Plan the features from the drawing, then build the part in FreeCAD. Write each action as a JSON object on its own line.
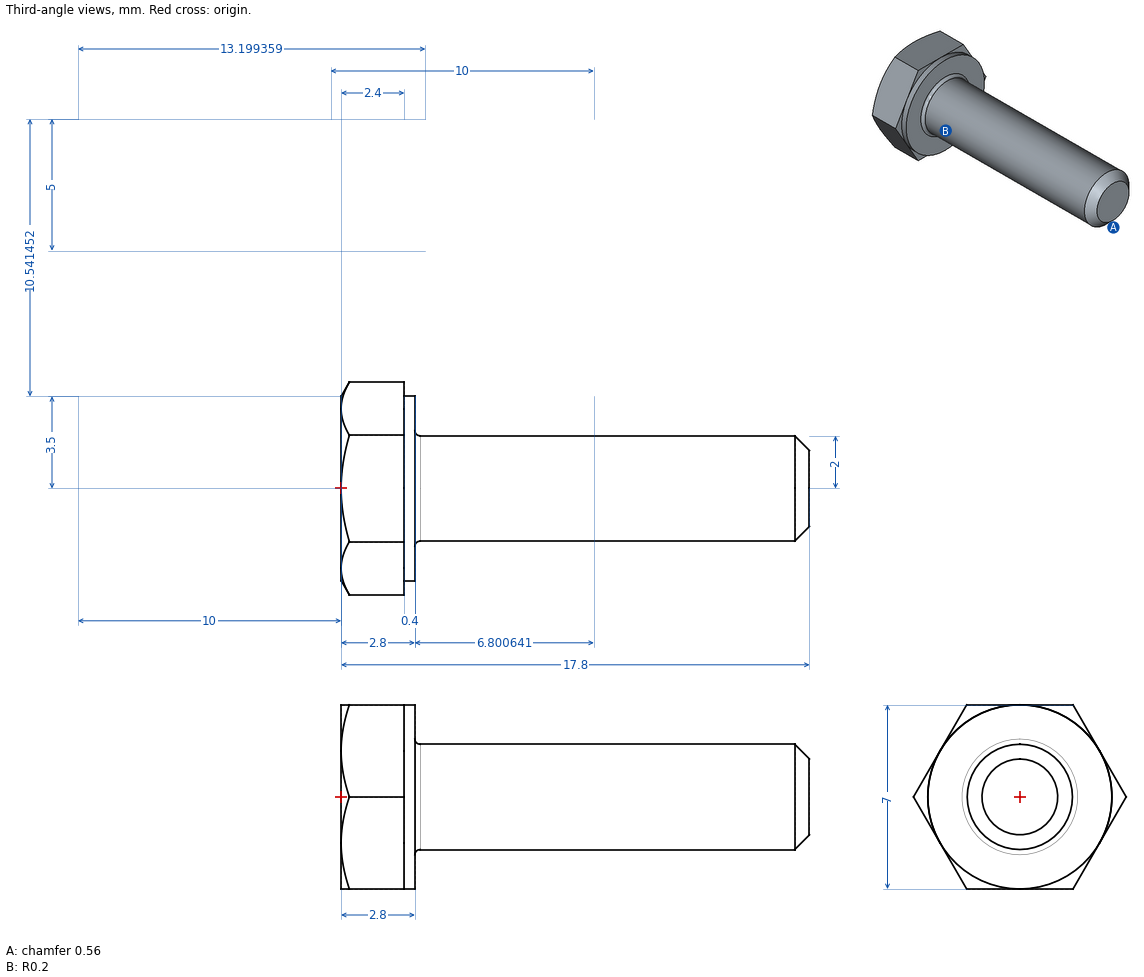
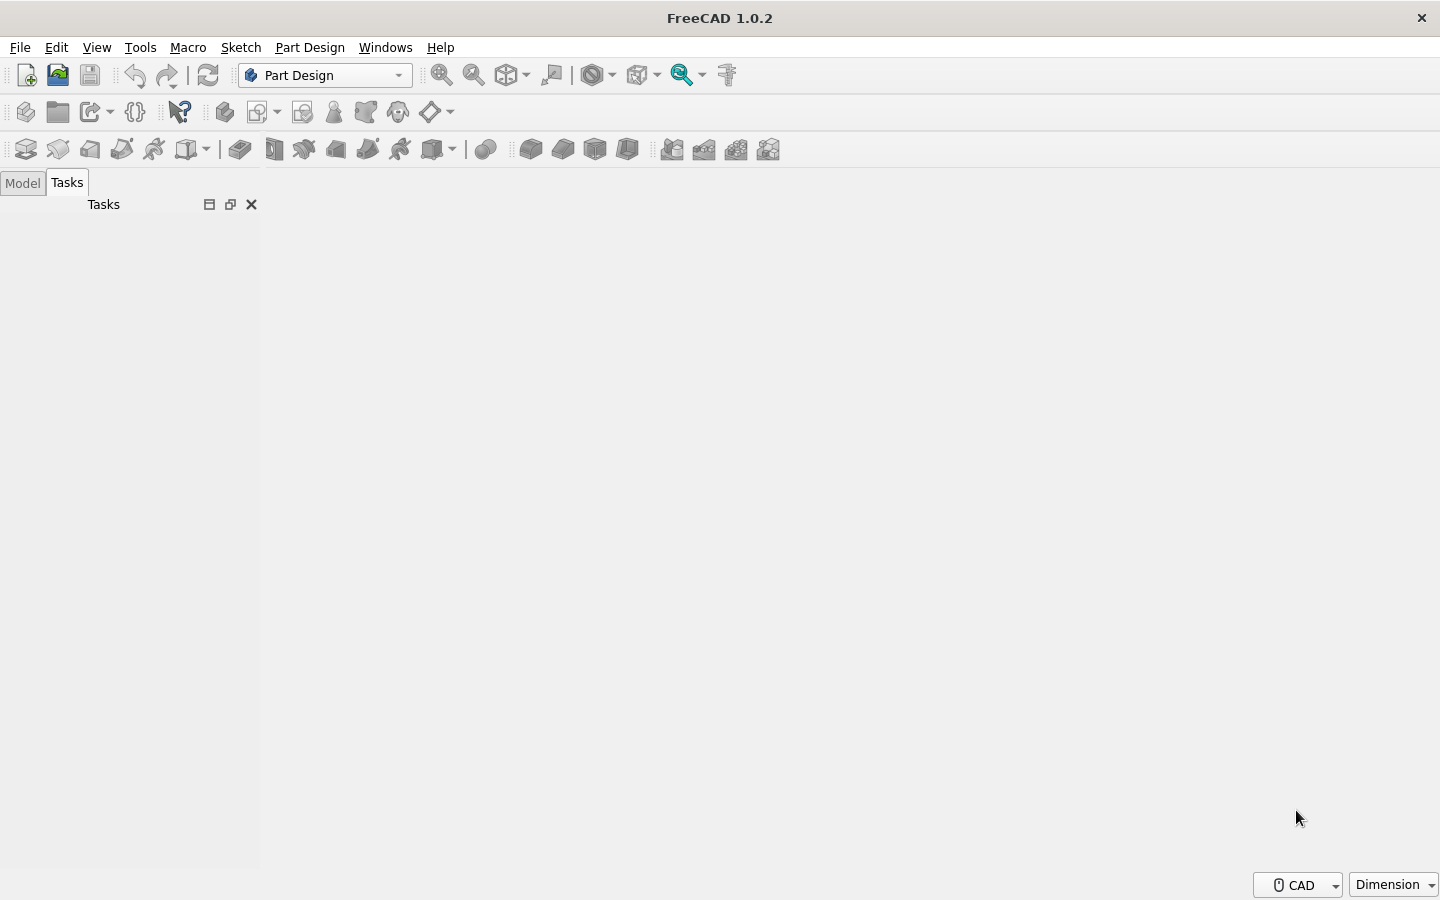
{"action": "key", "text": "ctrl+n"}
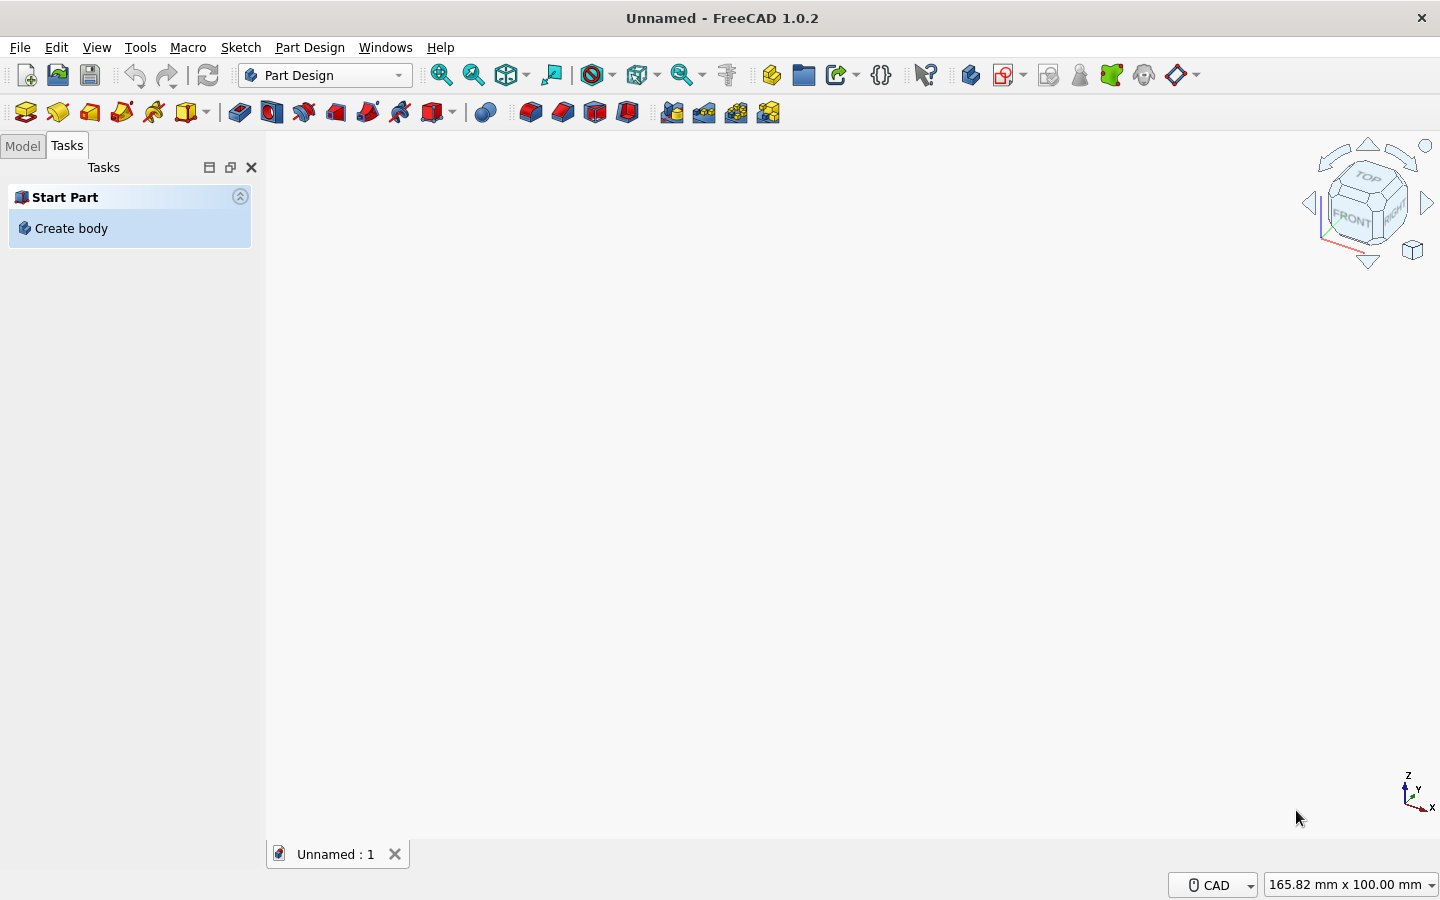
{"action": "left_click", "coordinate": [1004, 76]}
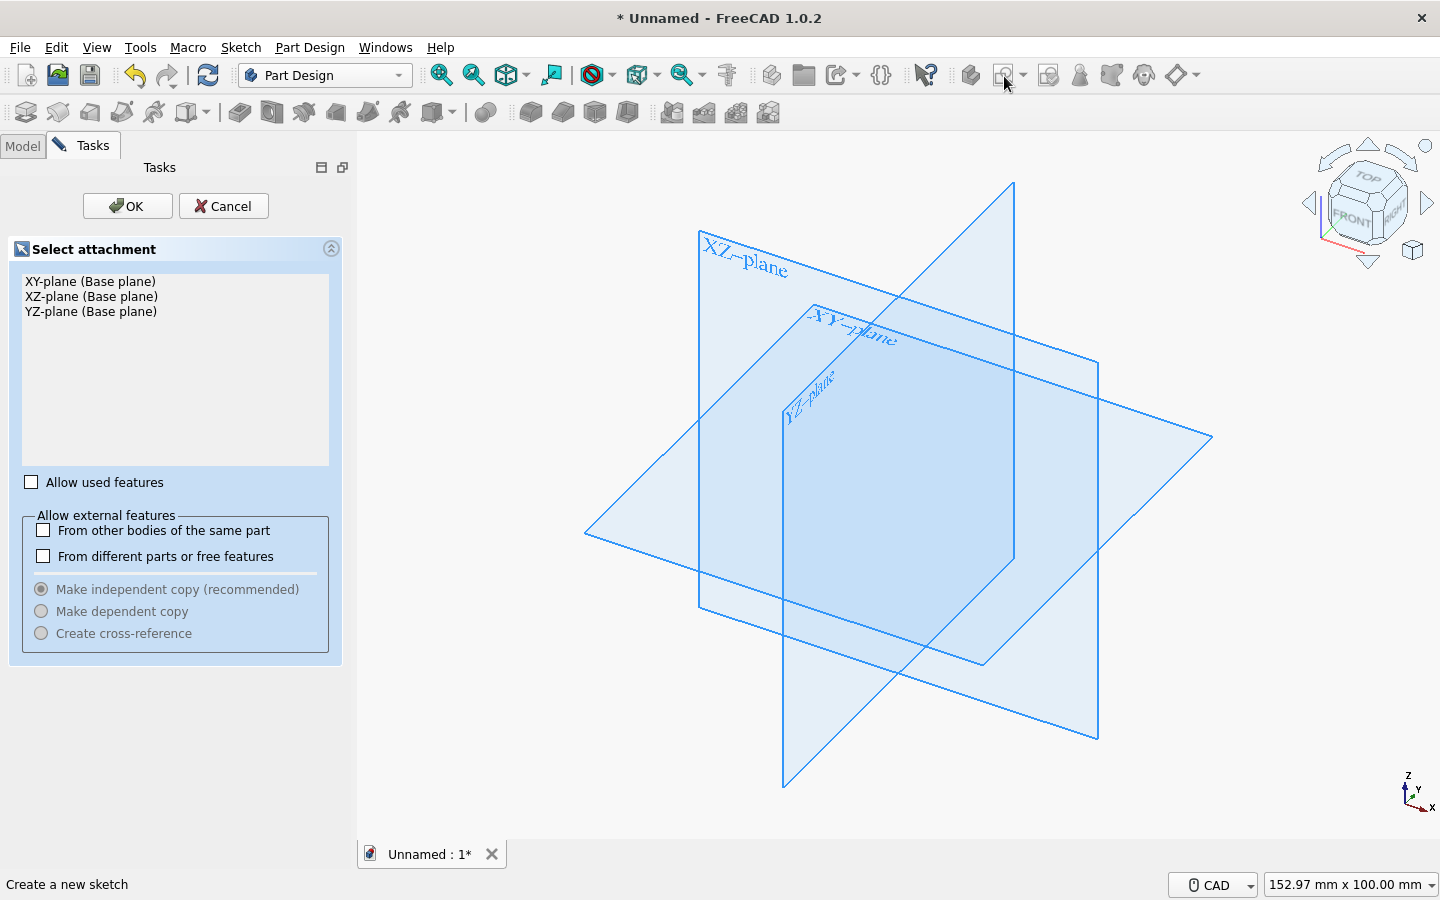
{"action": "left_click", "coordinate": [82, 312]}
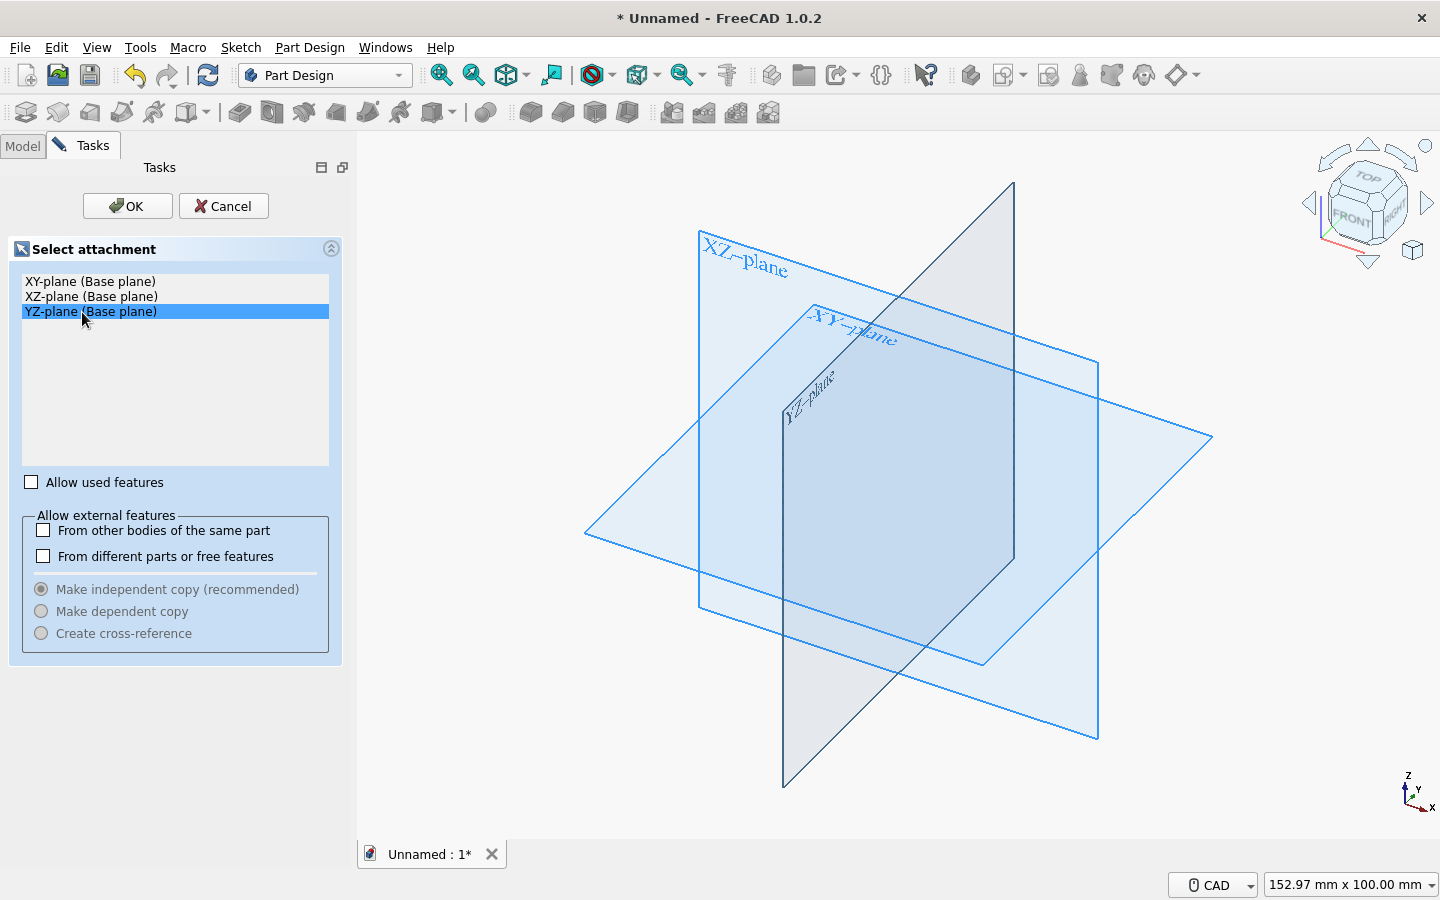
{"action": "left_click", "coordinate": [128, 206]}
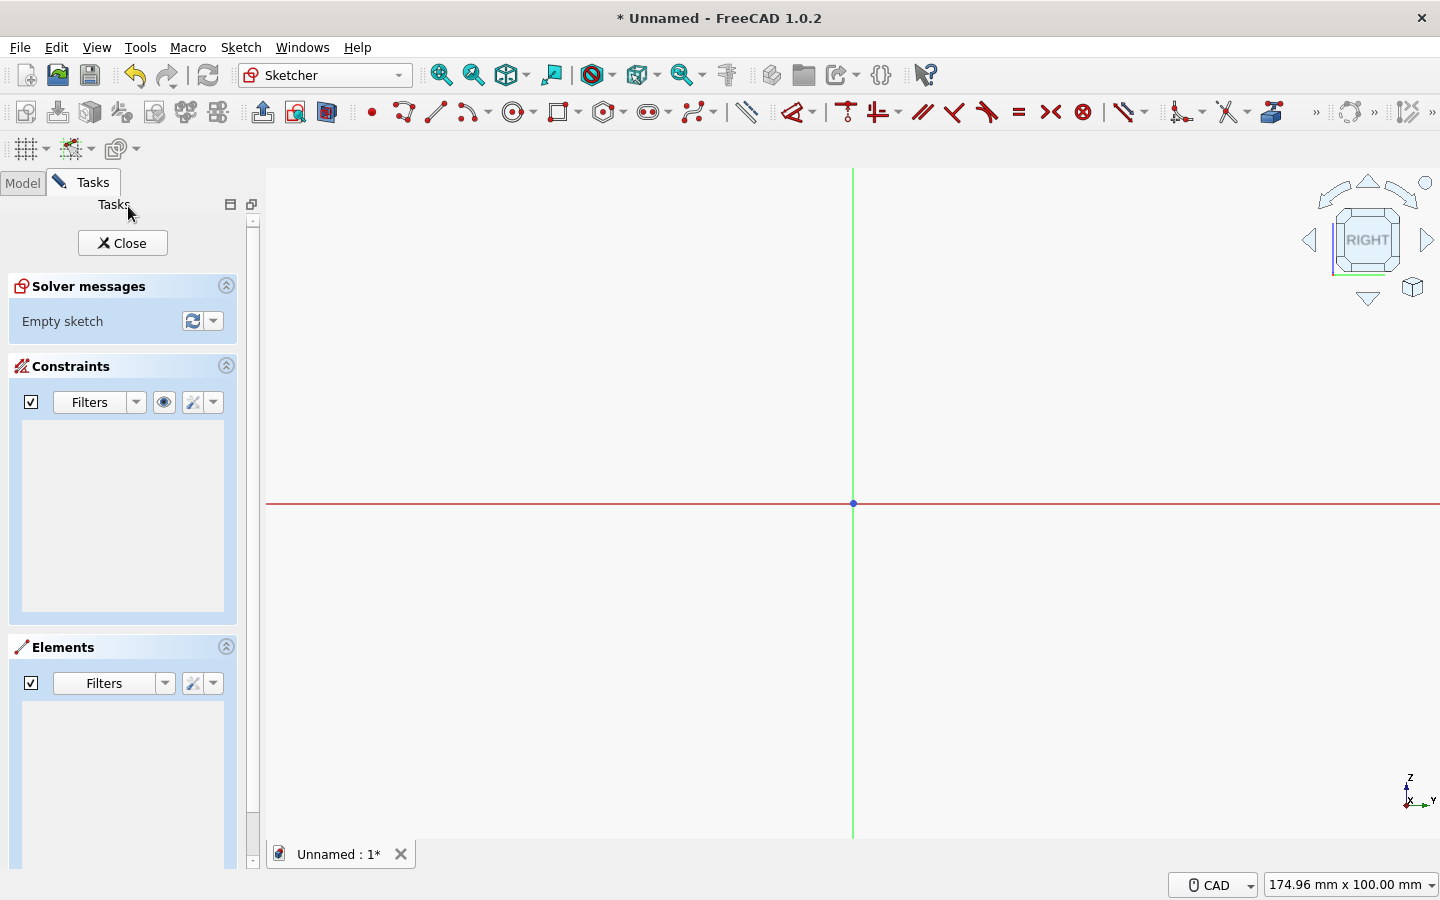
{"action": "scroll", "coordinate": [862, 504], "scroll_direction": "up", "scroll_amount": 11}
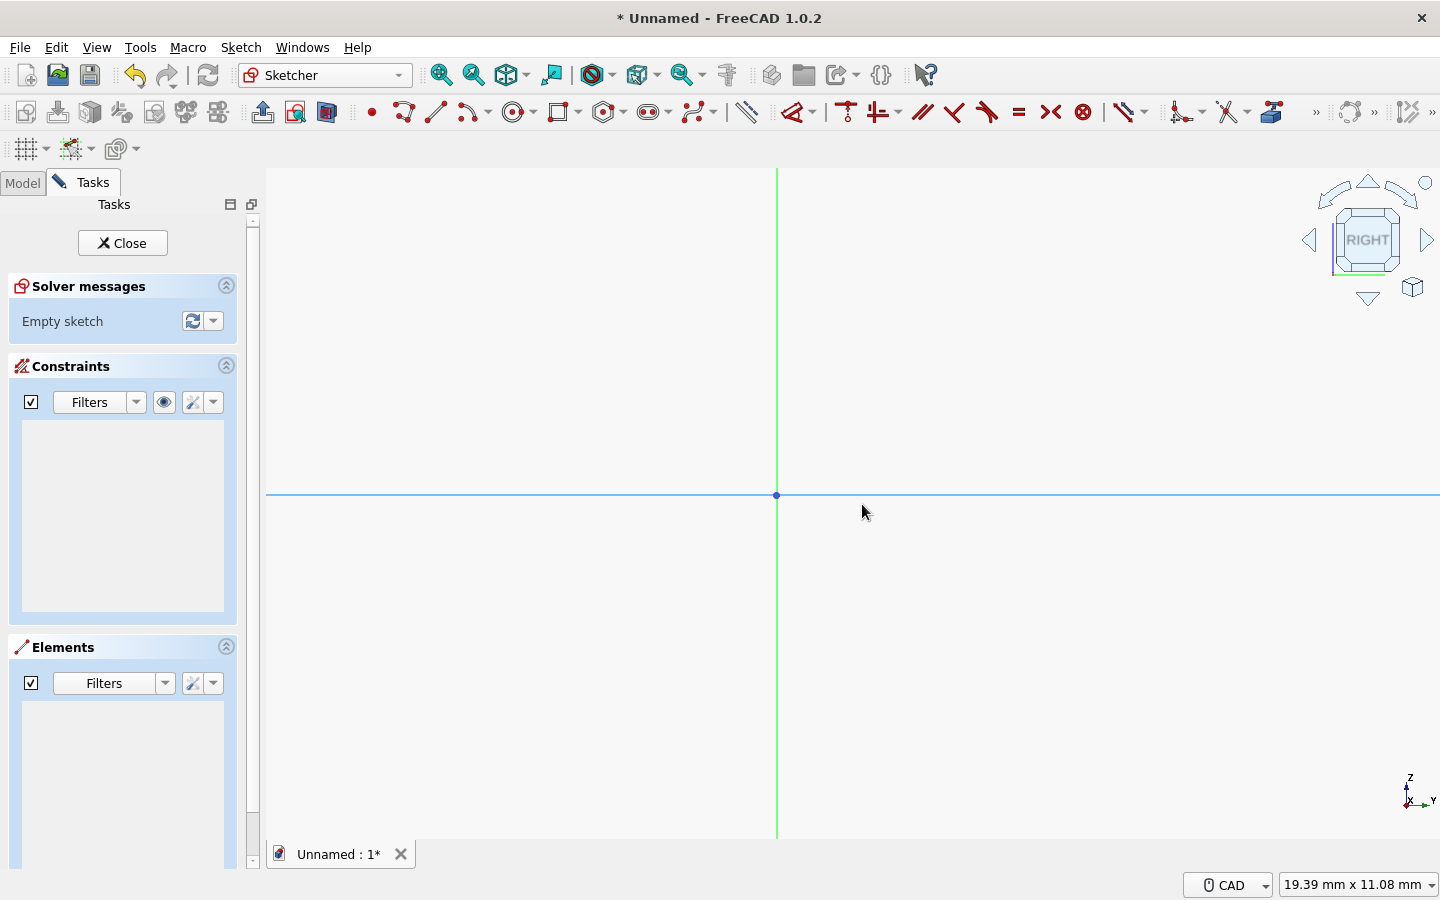
{"action": "key", "text": "g p 6"}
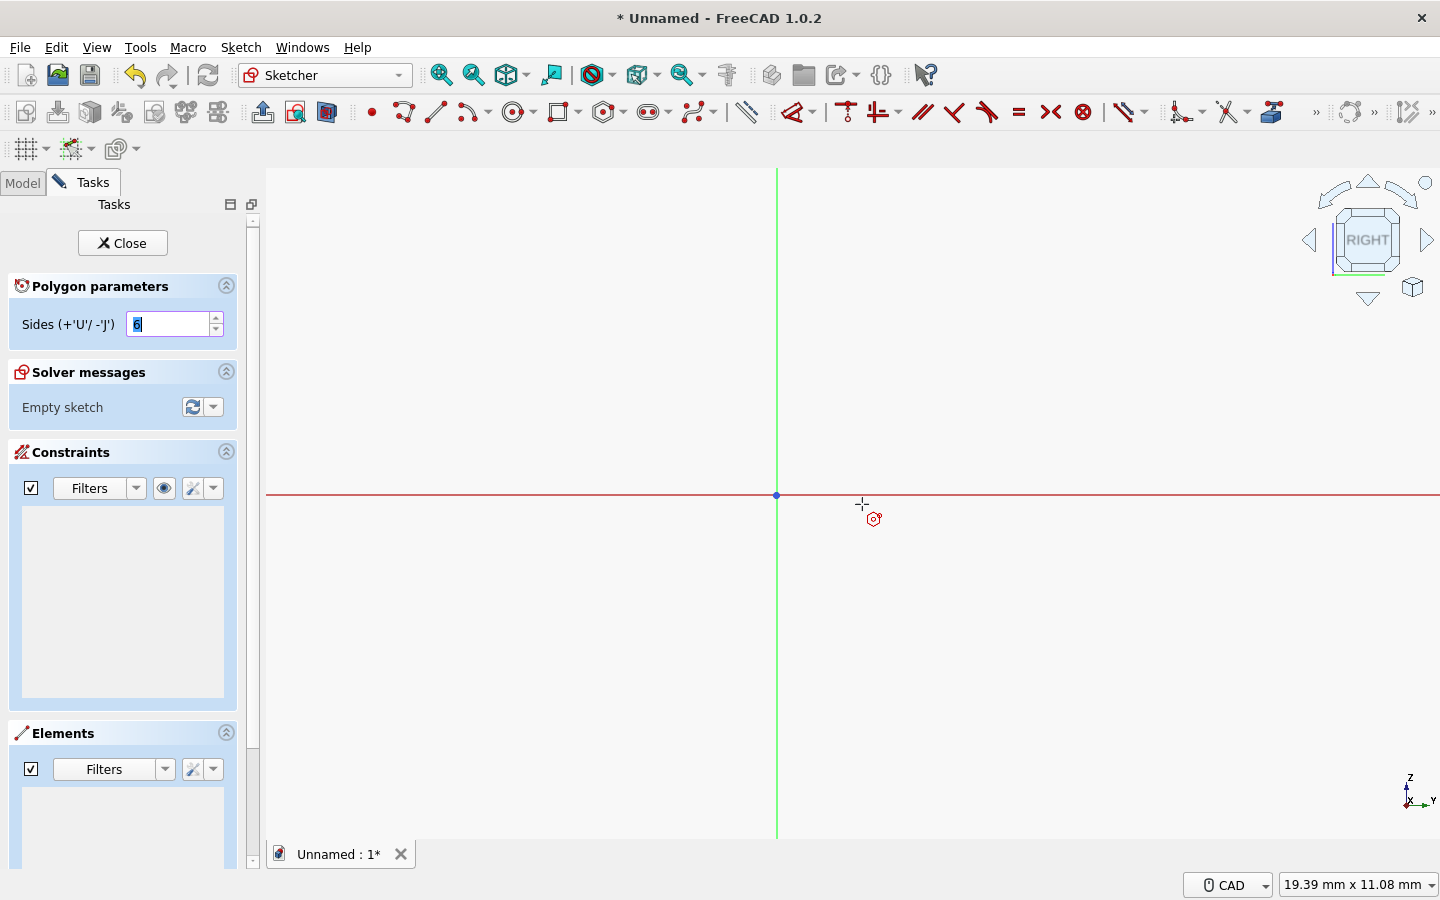
{"action": "left_click", "coordinate": [777, 495]}